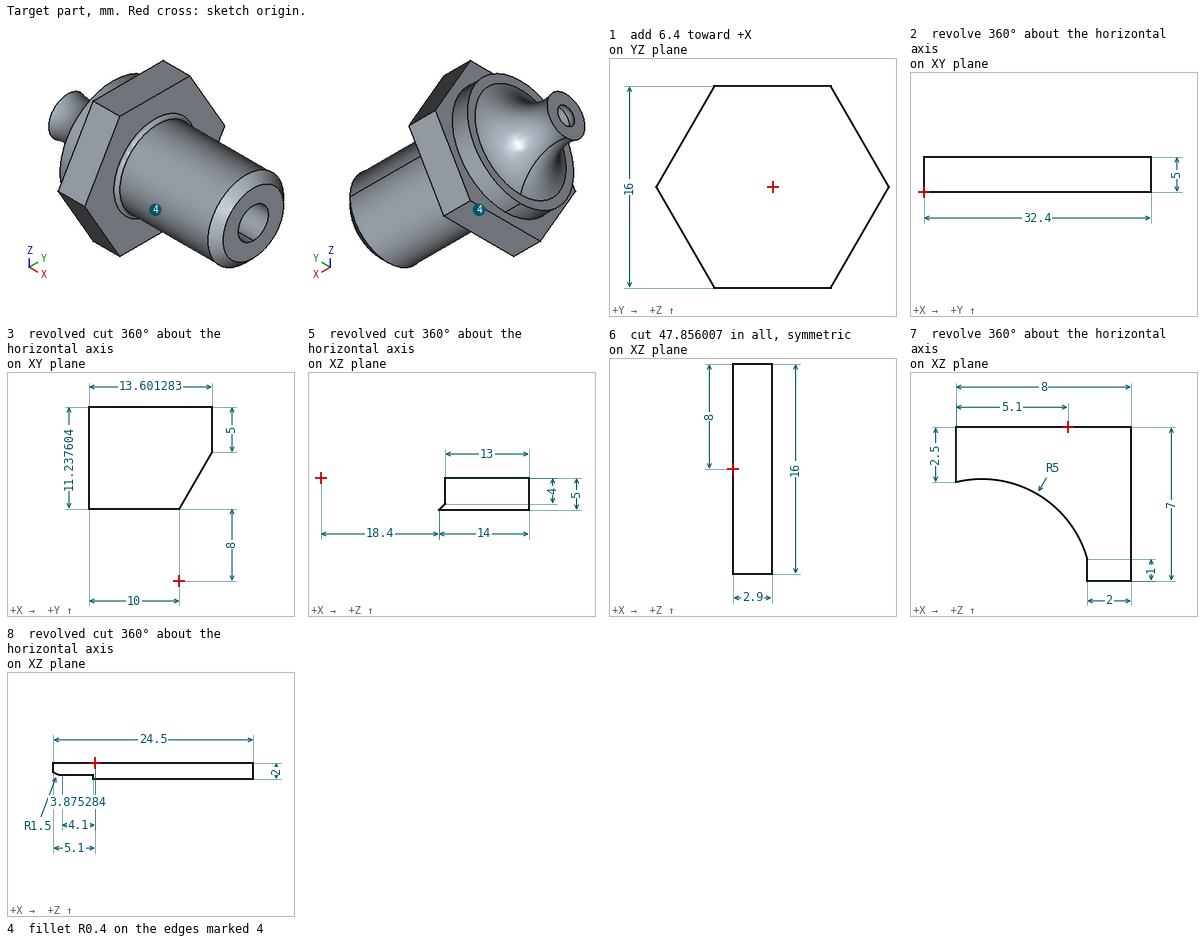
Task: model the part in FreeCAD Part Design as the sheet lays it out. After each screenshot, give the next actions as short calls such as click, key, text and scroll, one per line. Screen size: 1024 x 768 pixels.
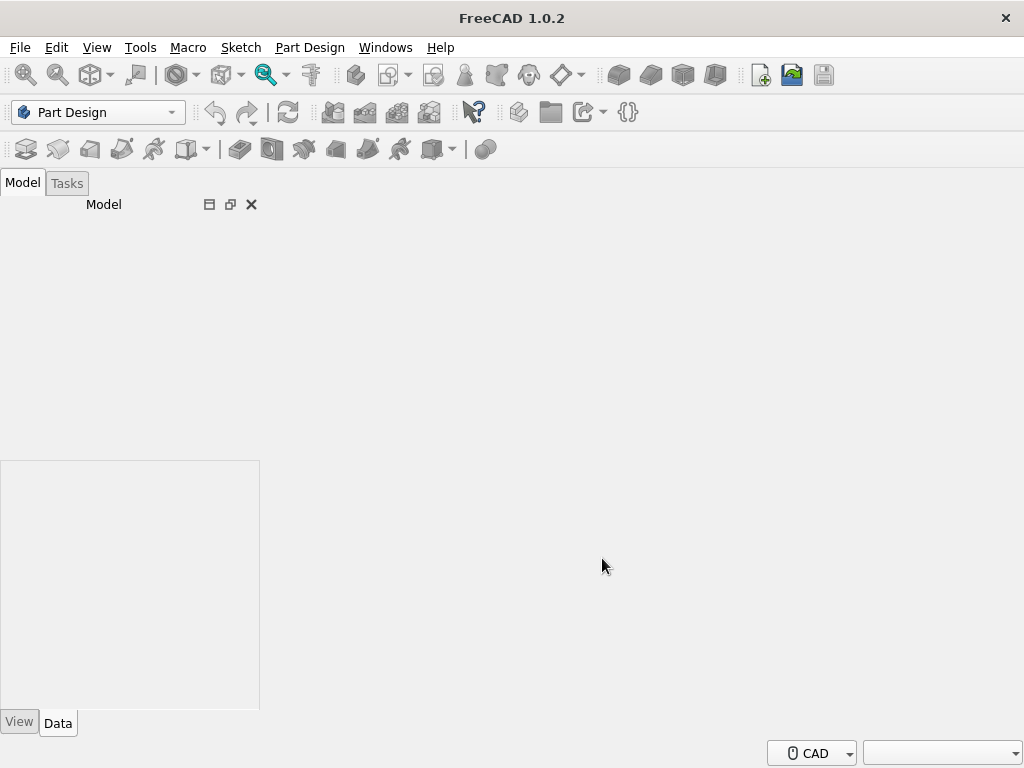
click(760, 76)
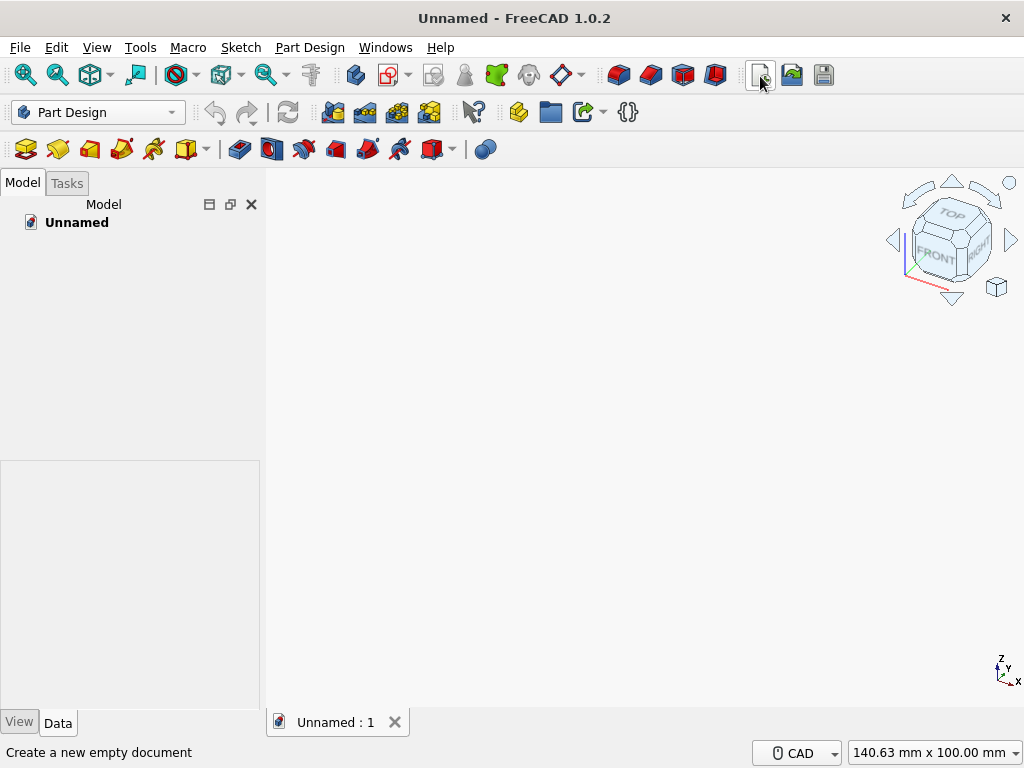
click(388, 76)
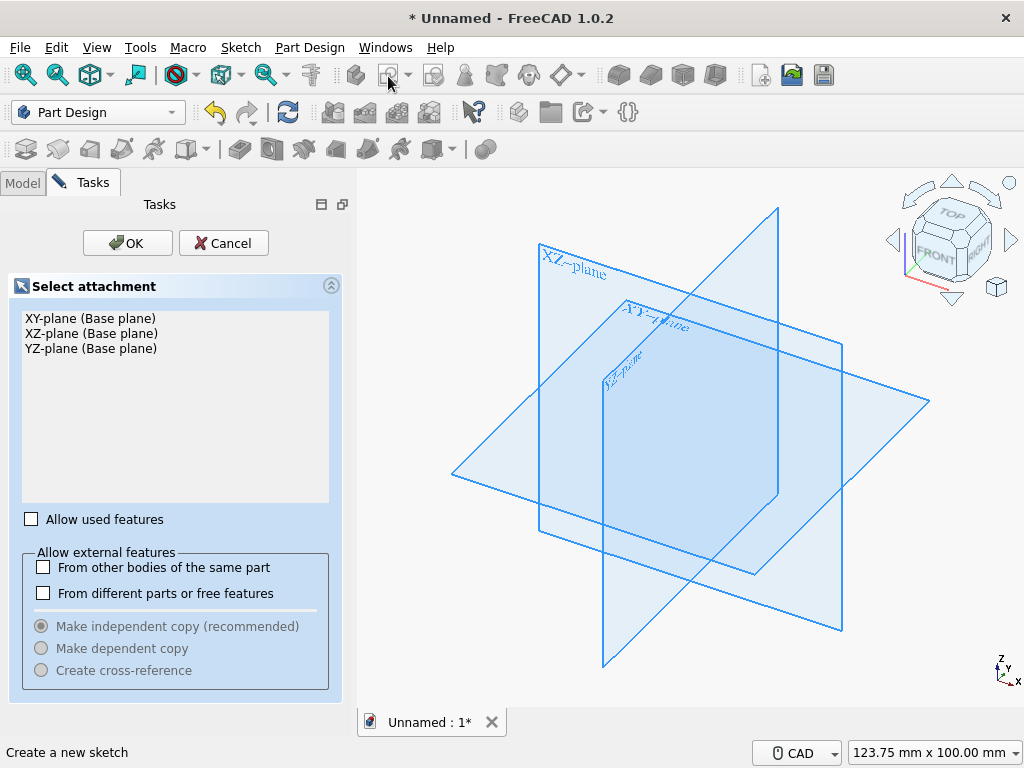
click(82, 348)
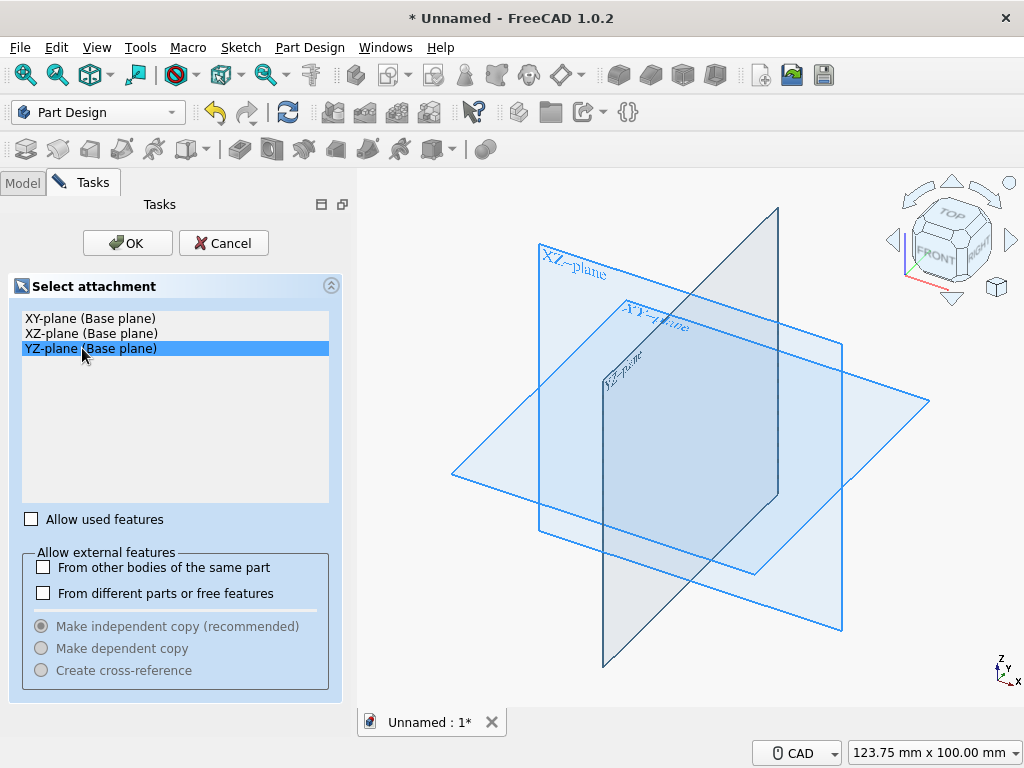
click(128, 243)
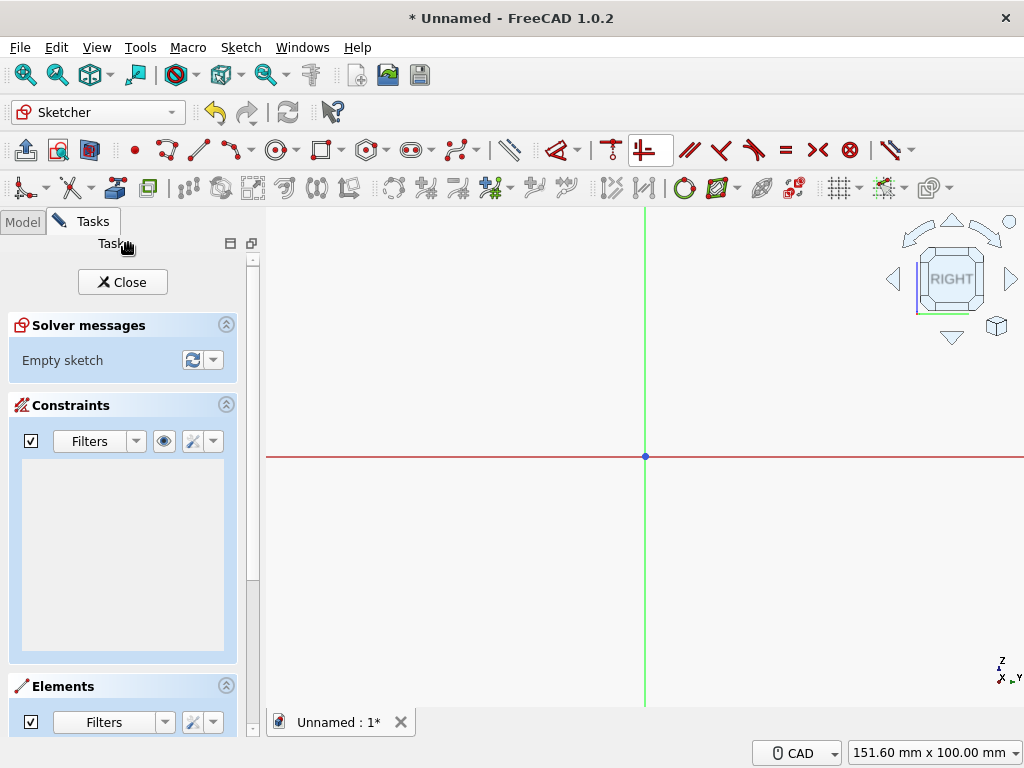
scroll(667, 457, up, 7)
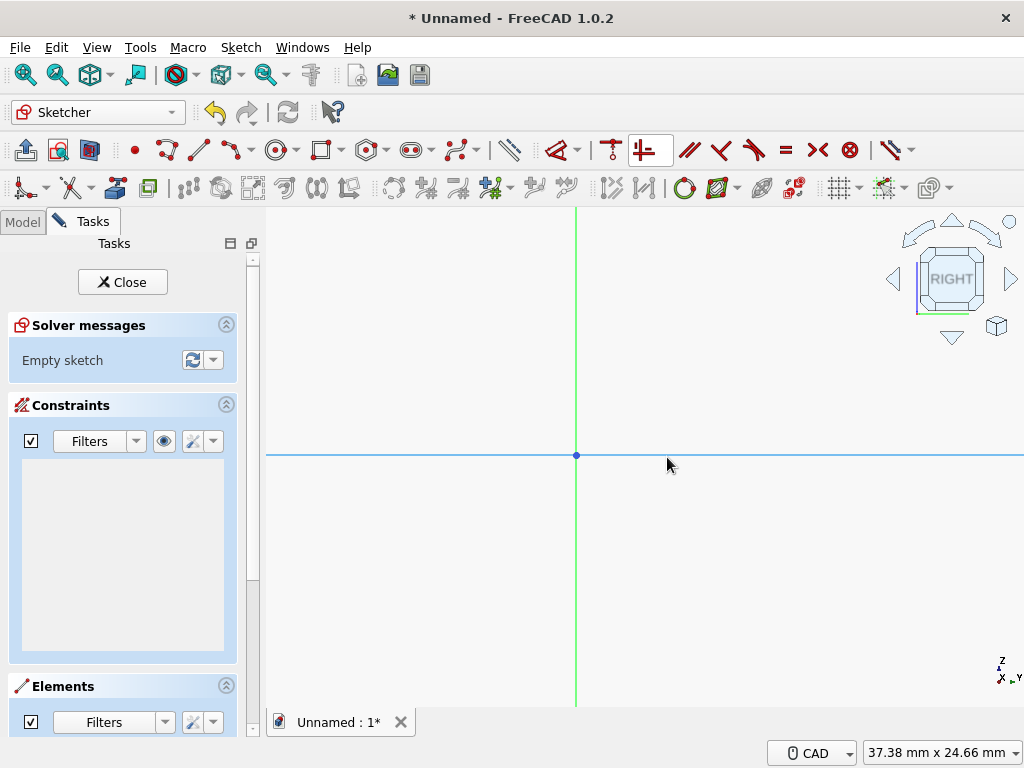
click(366, 150)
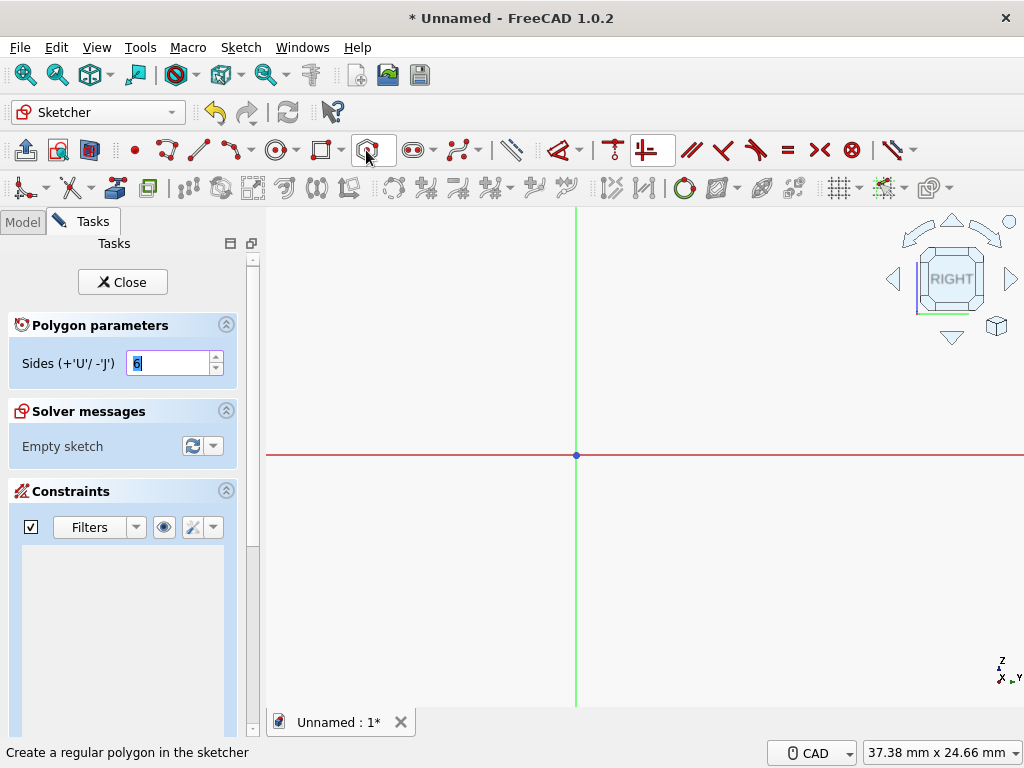
click(576, 455)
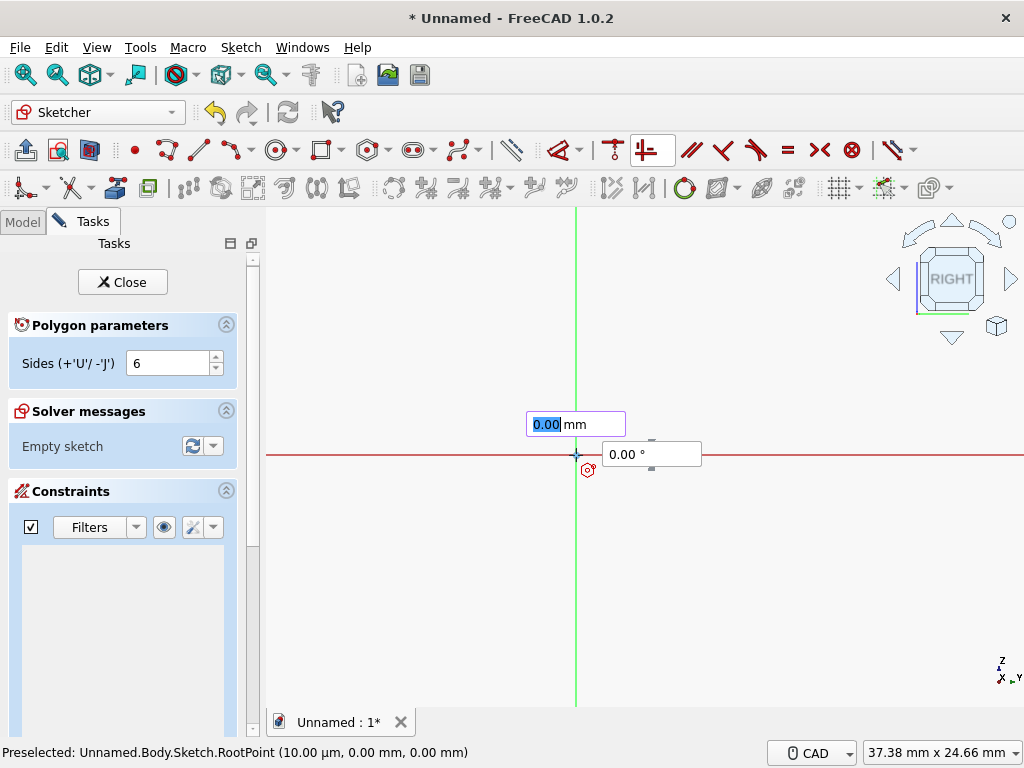
click(763, 455)
right_click(763, 455)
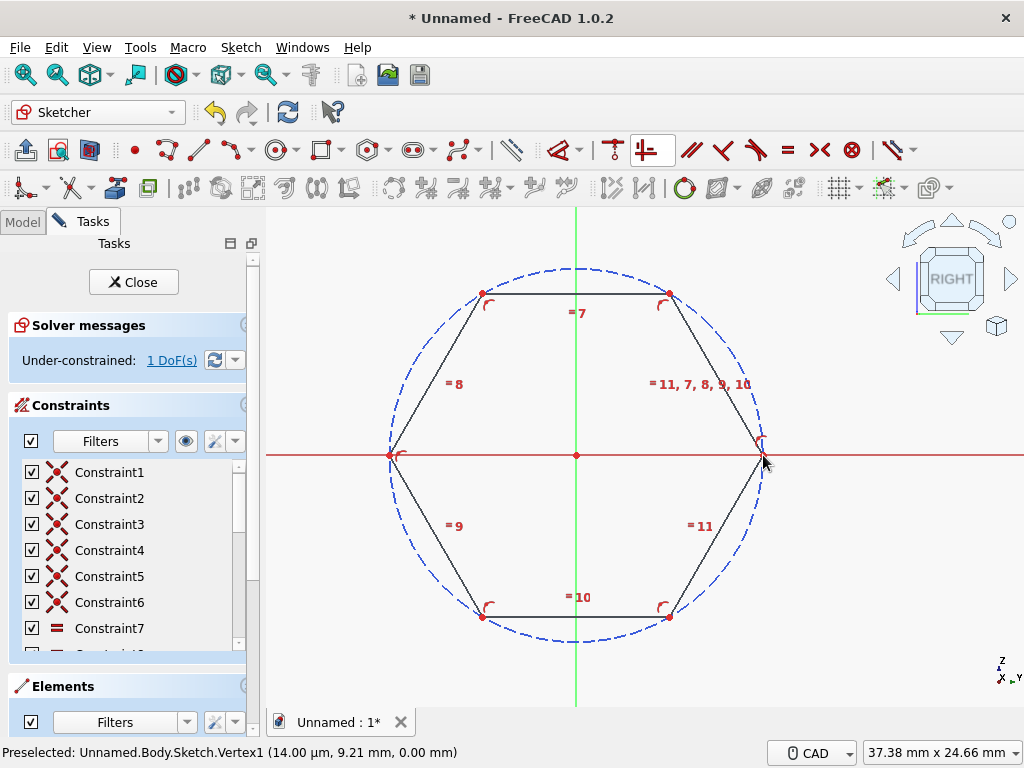
click(558, 150)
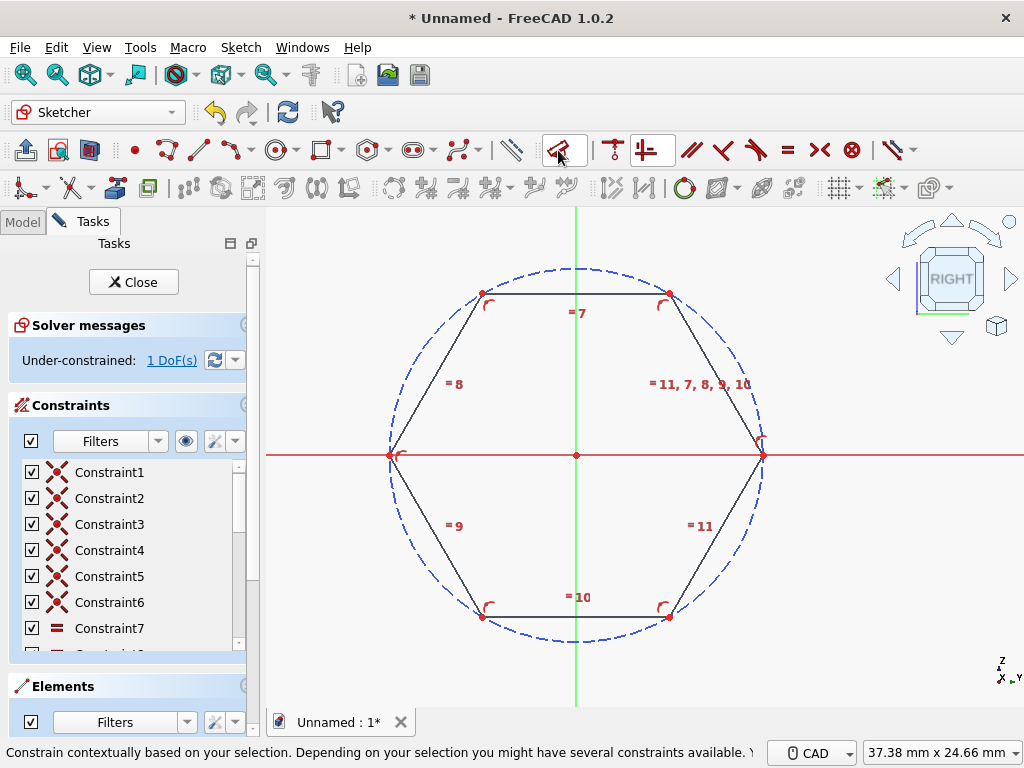
click(483, 617)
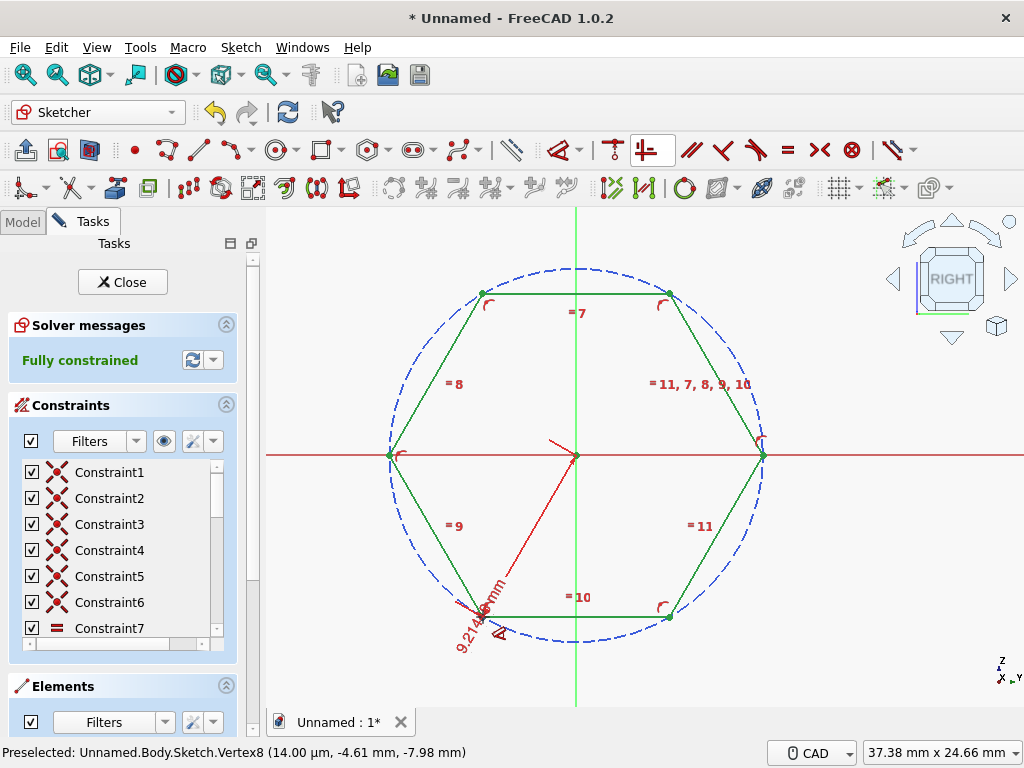
click(670, 294)
click(704, 381)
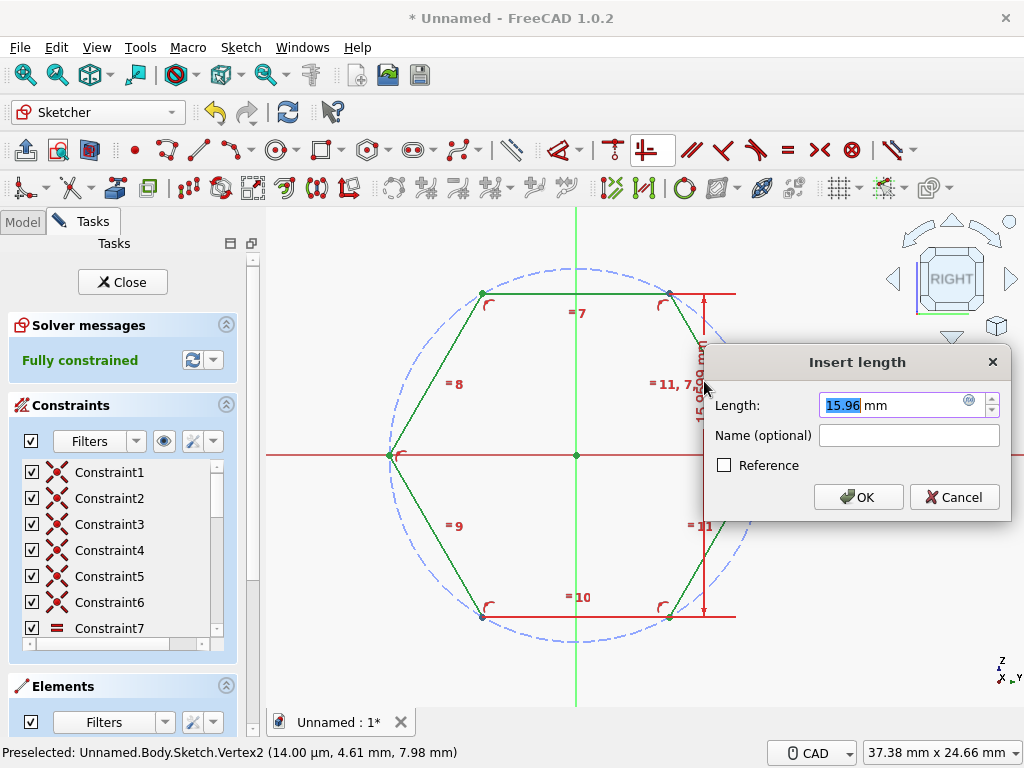
text(16)
key(Return)
key(Escape)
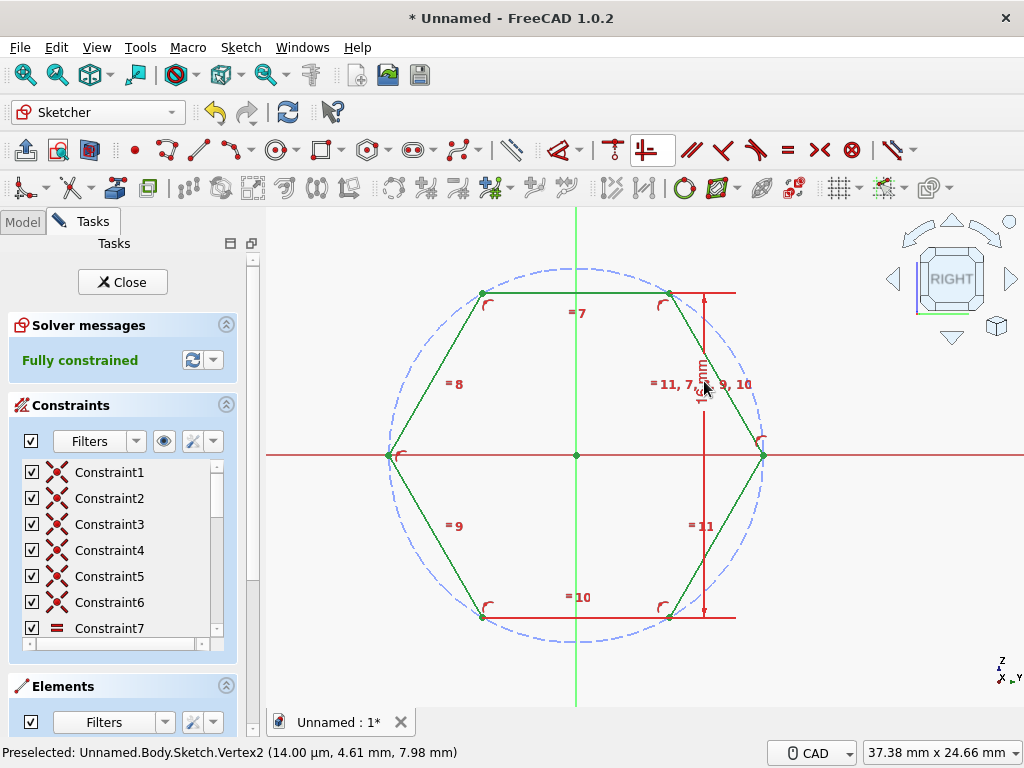
click(123, 282)